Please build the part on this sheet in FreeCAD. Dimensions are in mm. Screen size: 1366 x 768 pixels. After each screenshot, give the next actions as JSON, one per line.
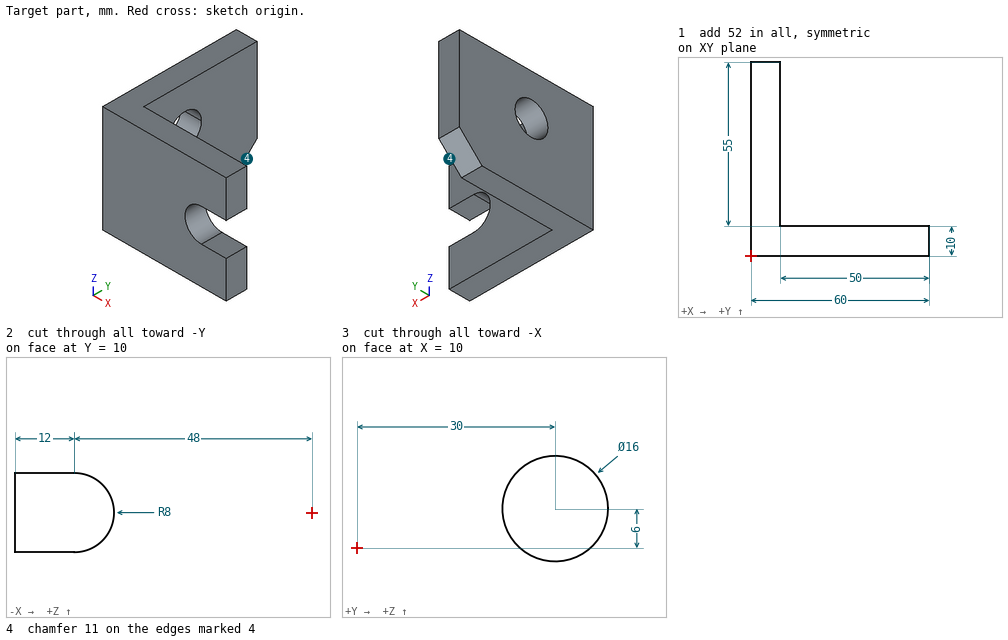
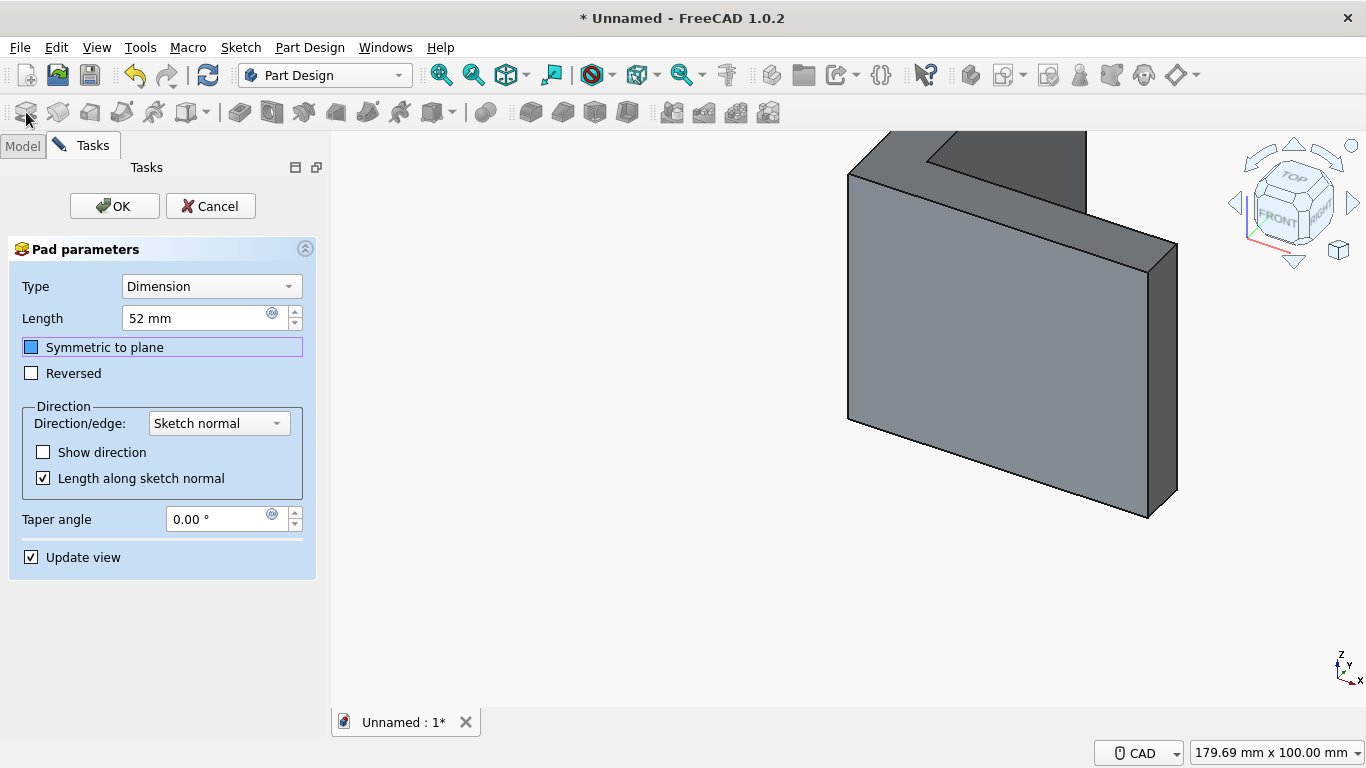
{"action": "left_click", "coordinate": [30, 347]}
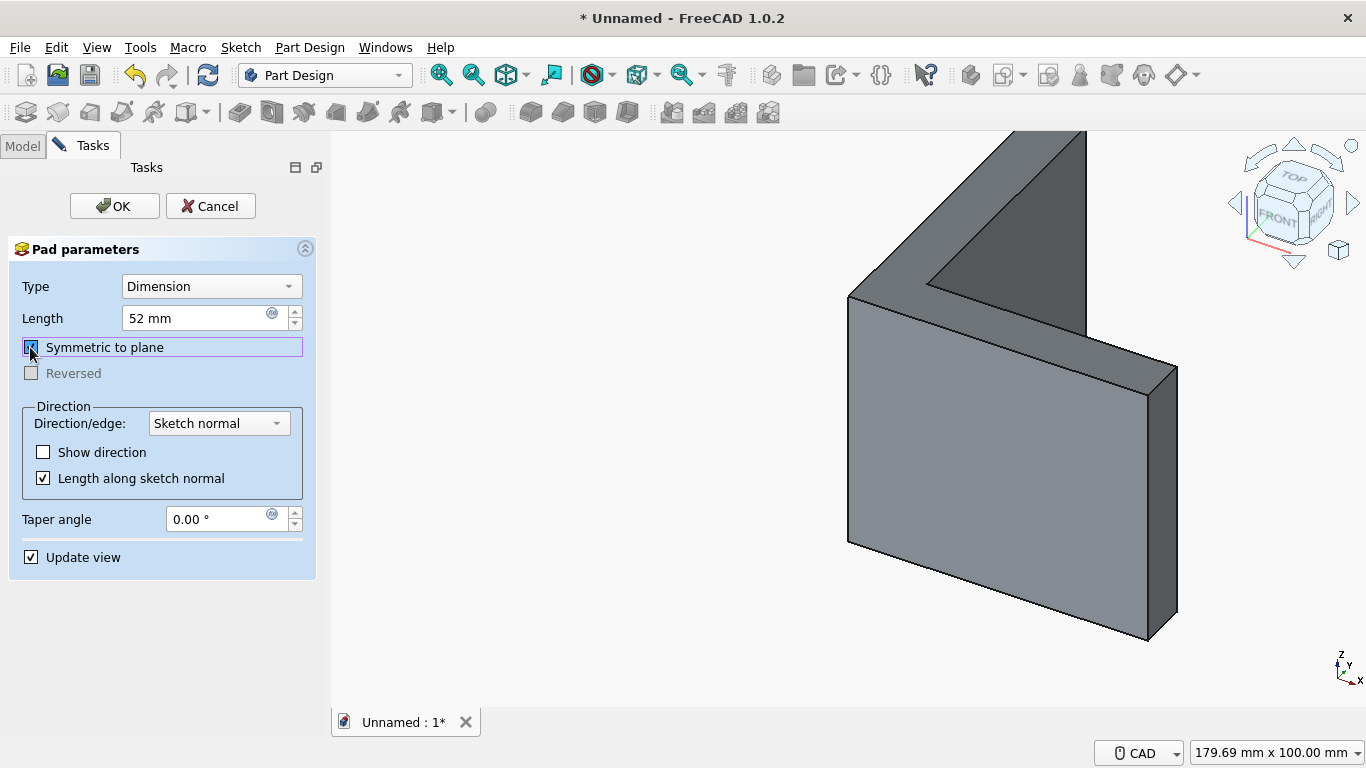
{"action": "left_click", "coordinate": [115, 206]}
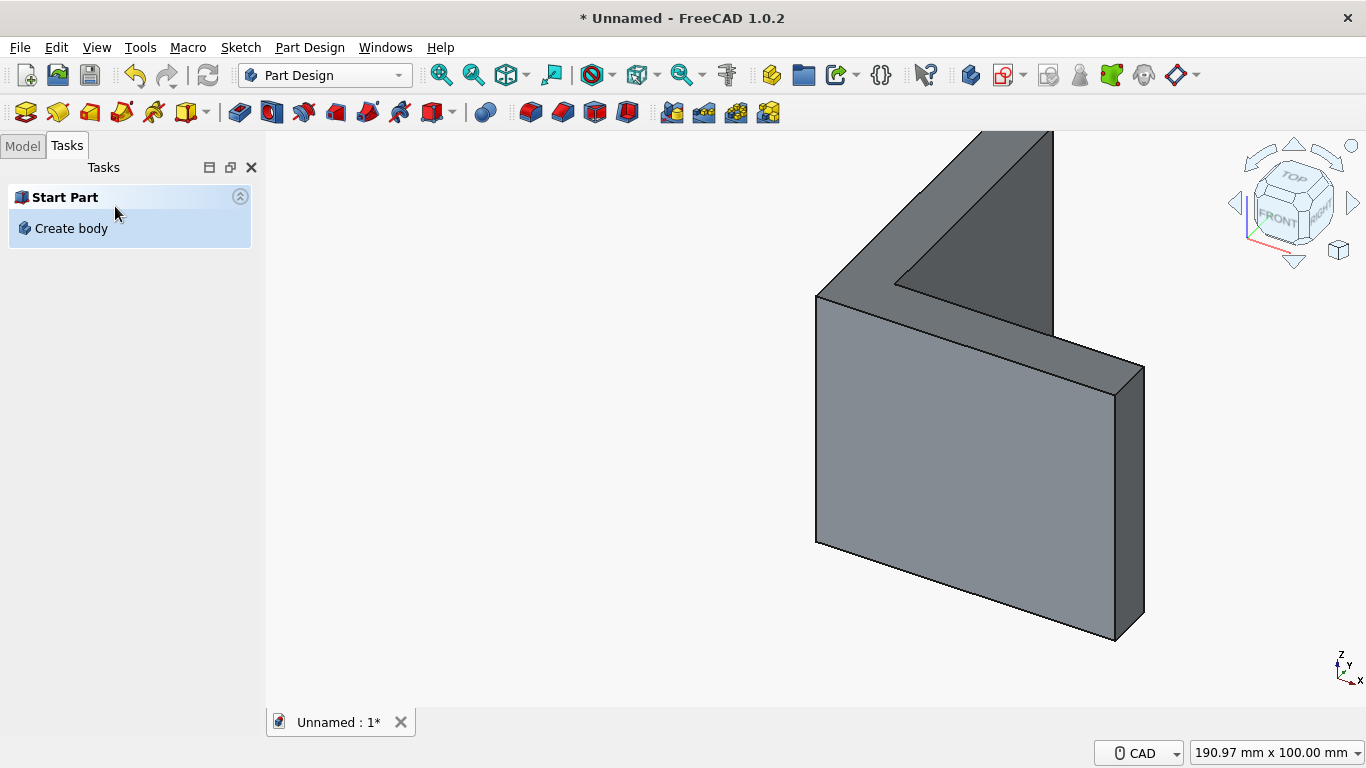
{"action": "left_click", "coordinate": [442, 76]}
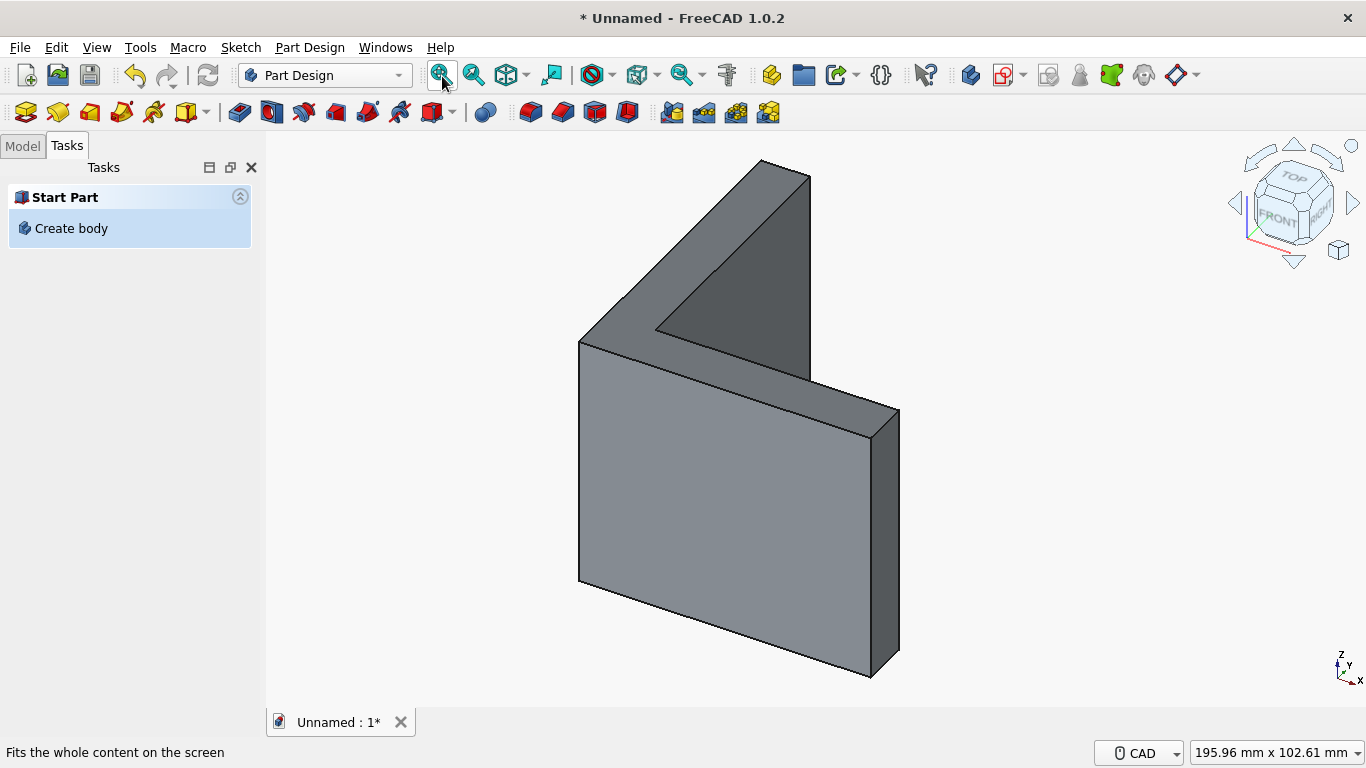
{"action": "key", "text": "4"}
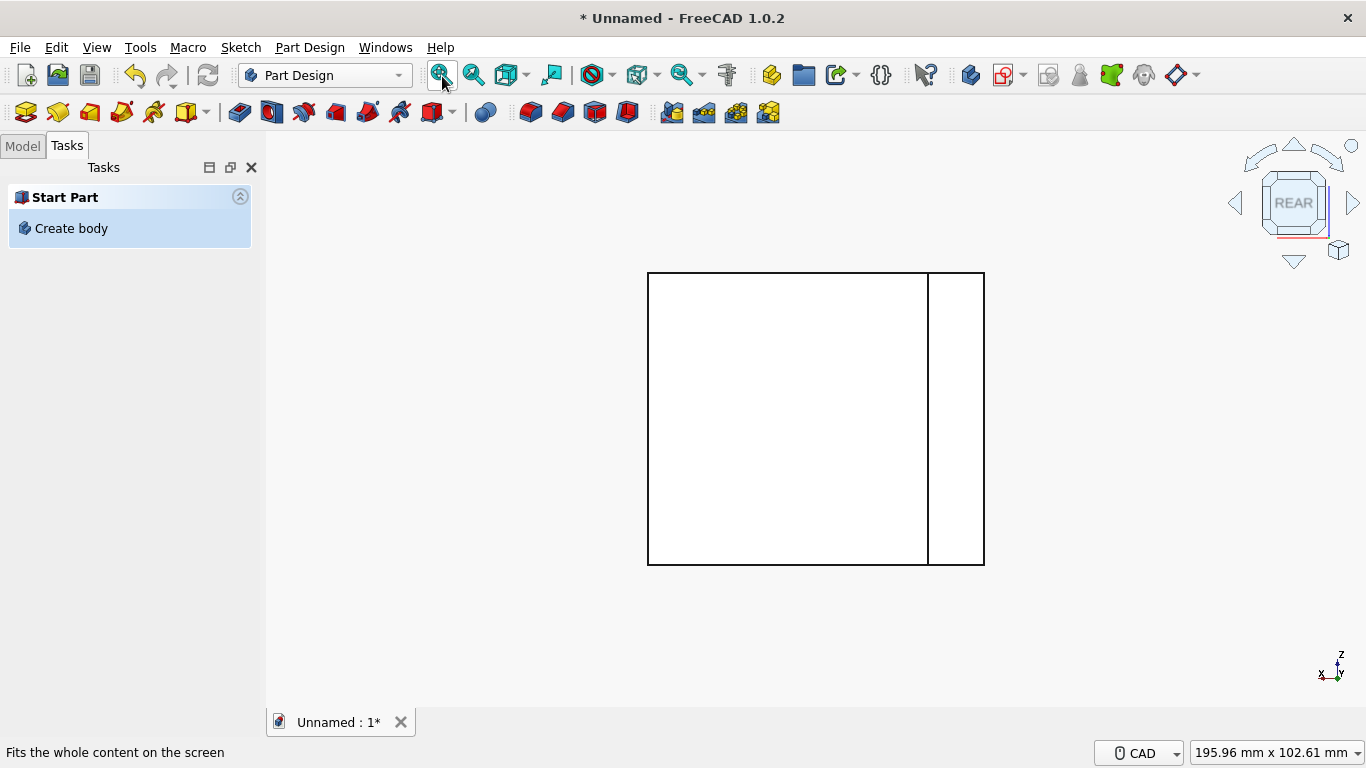
{"action": "left_click", "coordinate": [788, 418]}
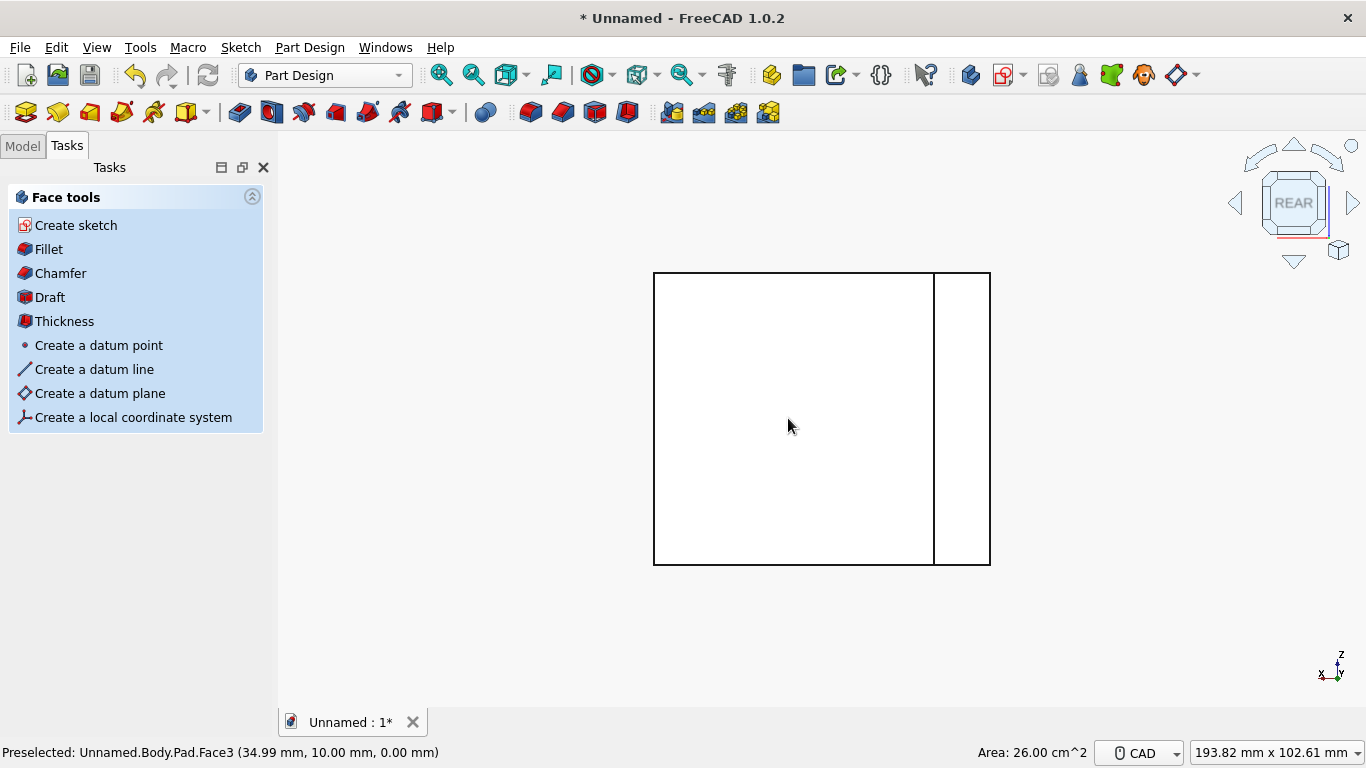
{"action": "left_click", "coordinate": [1004, 76]}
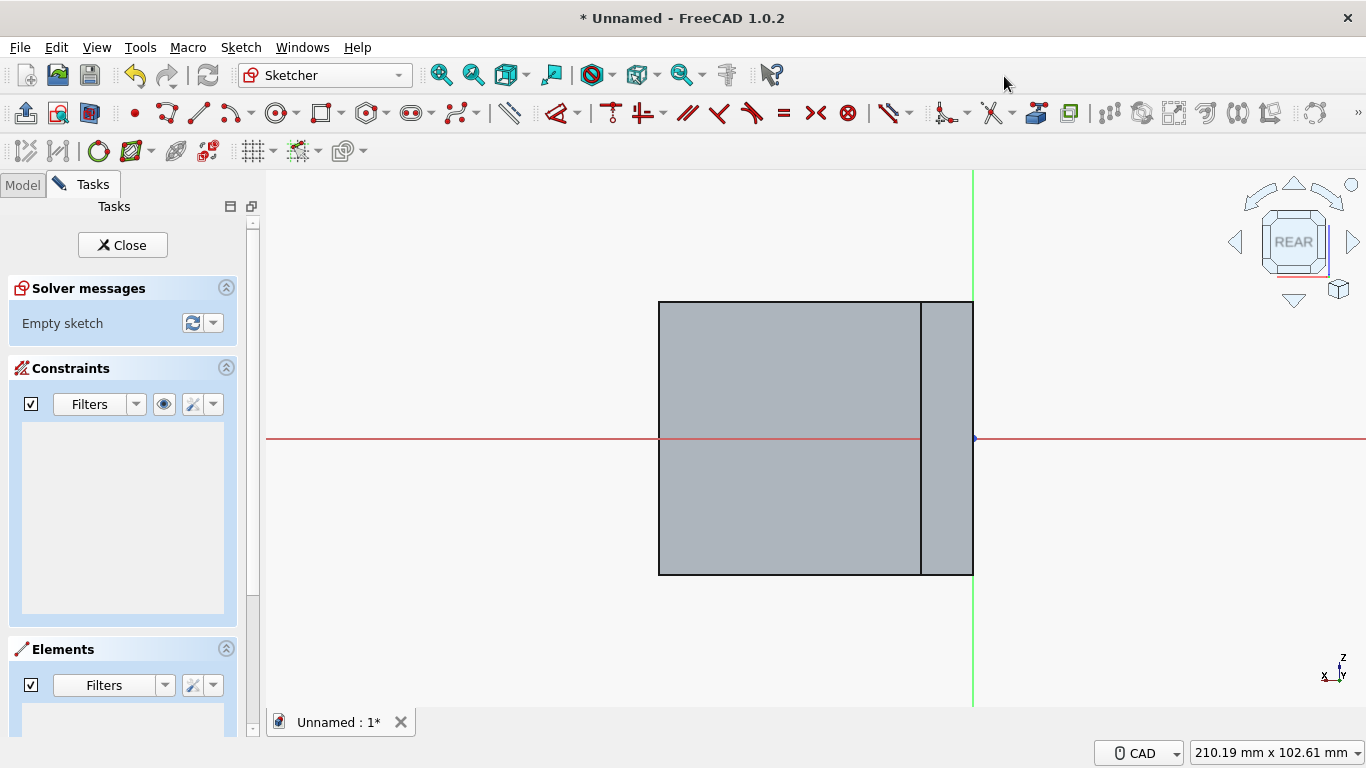
{"action": "left_click", "coordinate": [90, 114]}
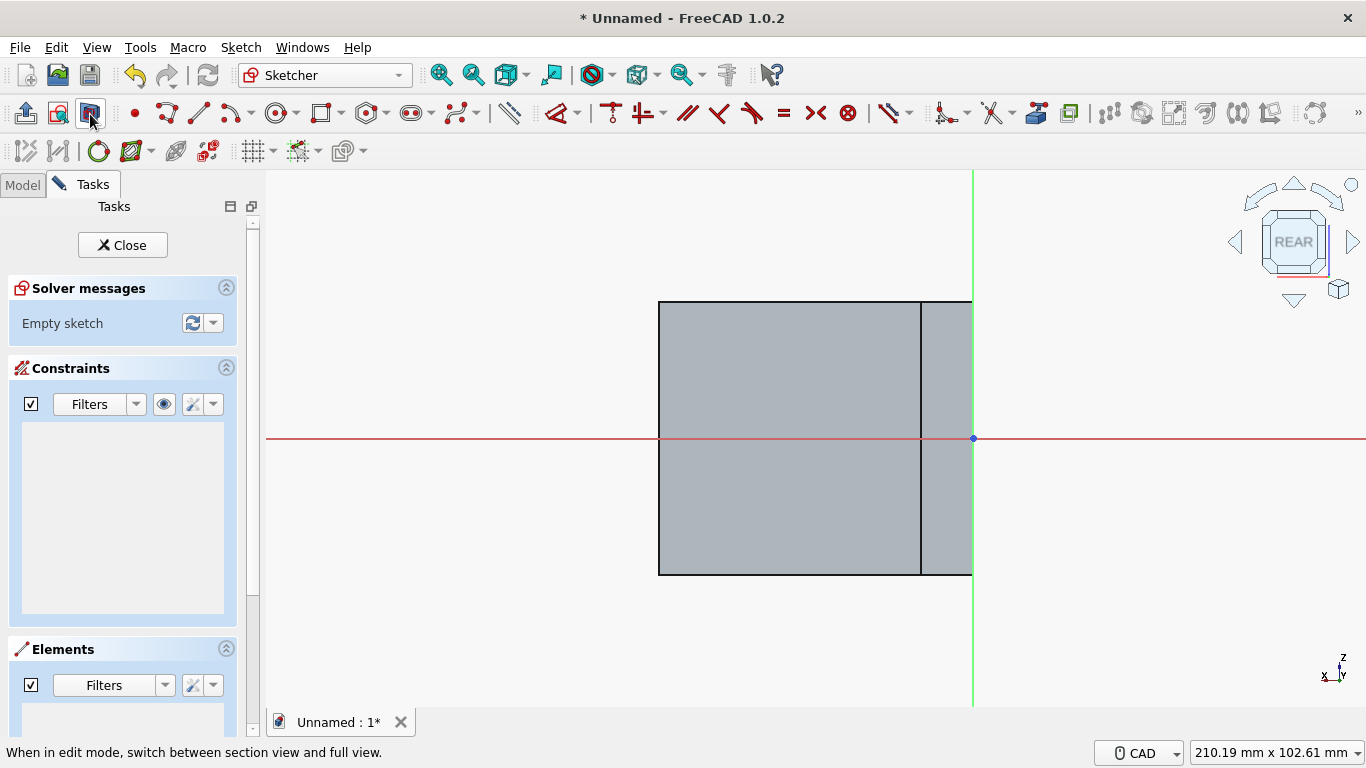
{"action": "scroll", "coordinate": [699, 438], "scroll_direction": "up", "scroll_amount": 7}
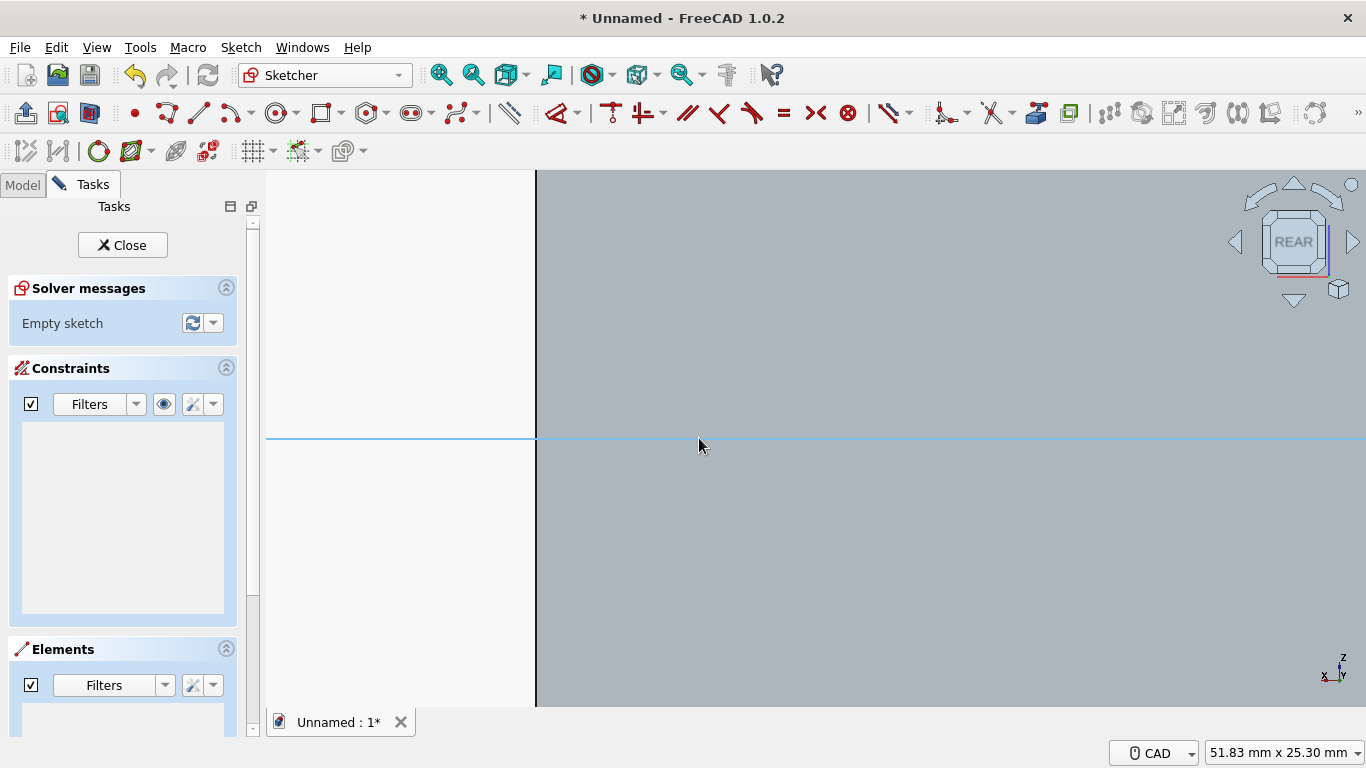
{"action": "left_click", "coordinate": [168, 114]}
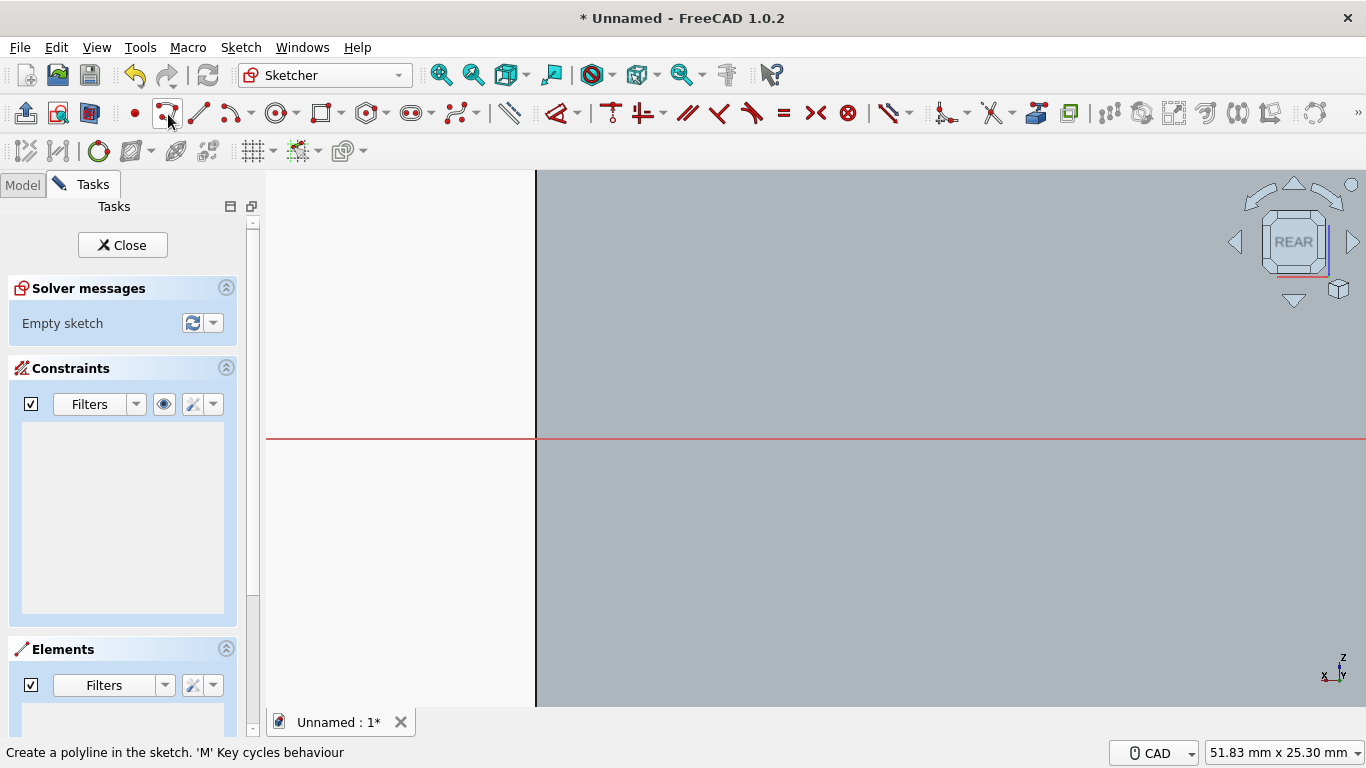
{"action": "left_click", "coordinate": [790, 269]}
{"action": "left_click", "coordinate": [536, 269]}
{"action": "left_click", "coordinate": [536, 608]}
{"action": "left_click", "coordinate": [790, 608]}
{"action": "right_click", "coordinate": [790, 608]}